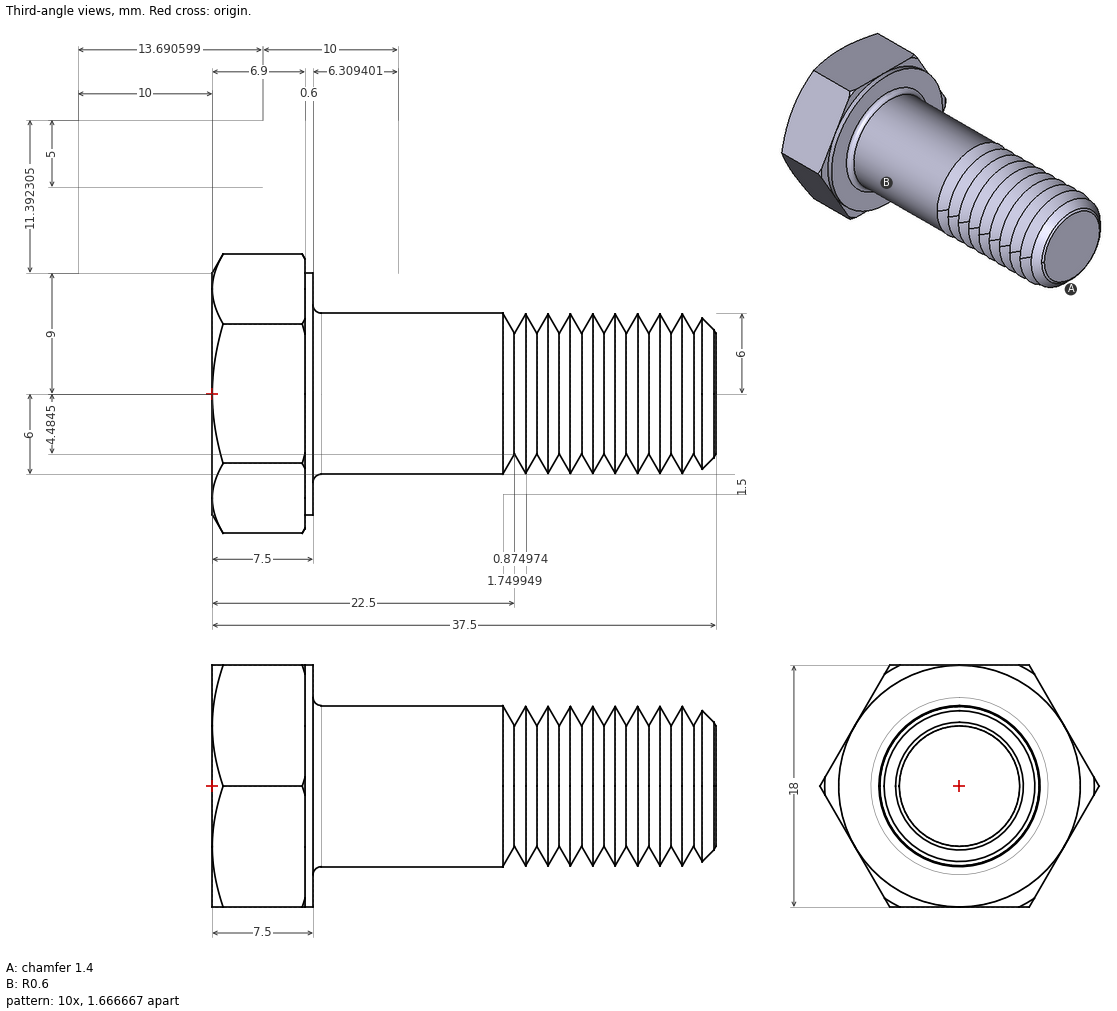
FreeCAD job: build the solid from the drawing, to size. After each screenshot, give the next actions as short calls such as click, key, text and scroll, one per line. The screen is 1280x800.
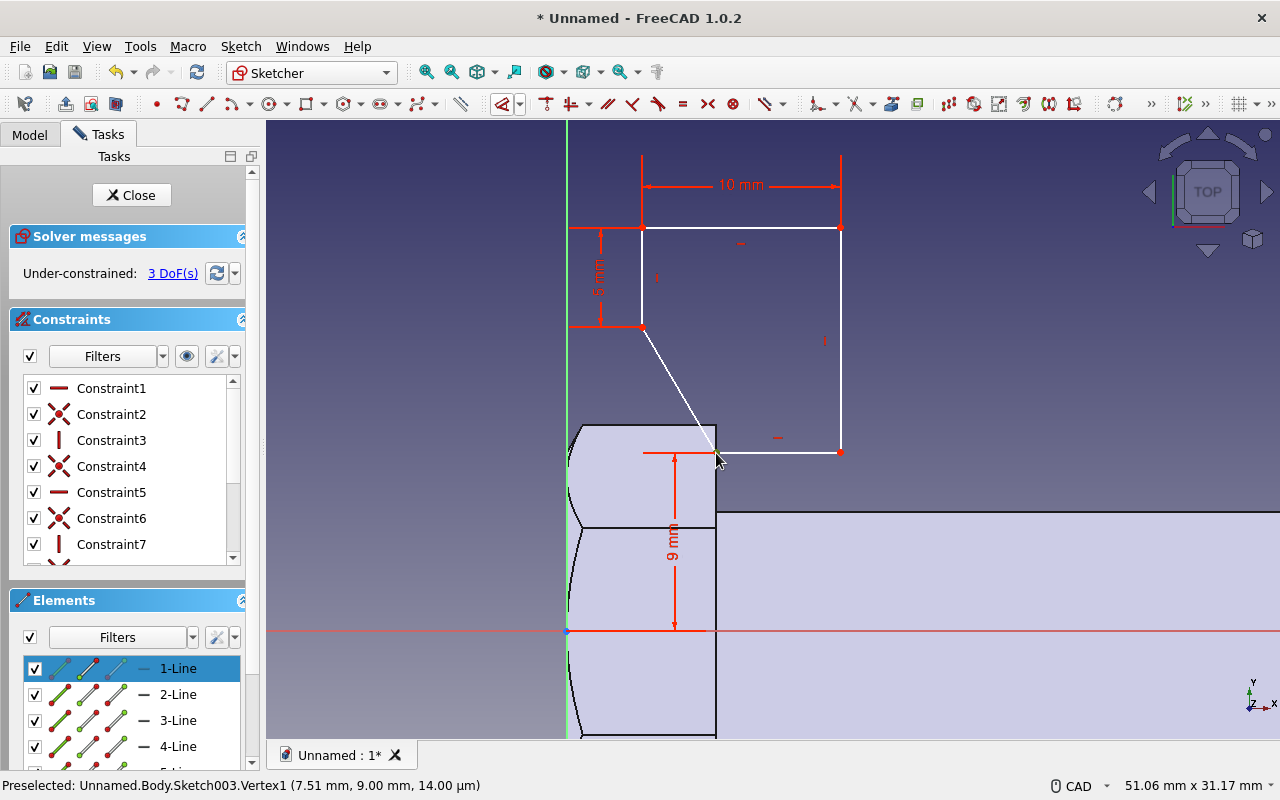
click(520, 104)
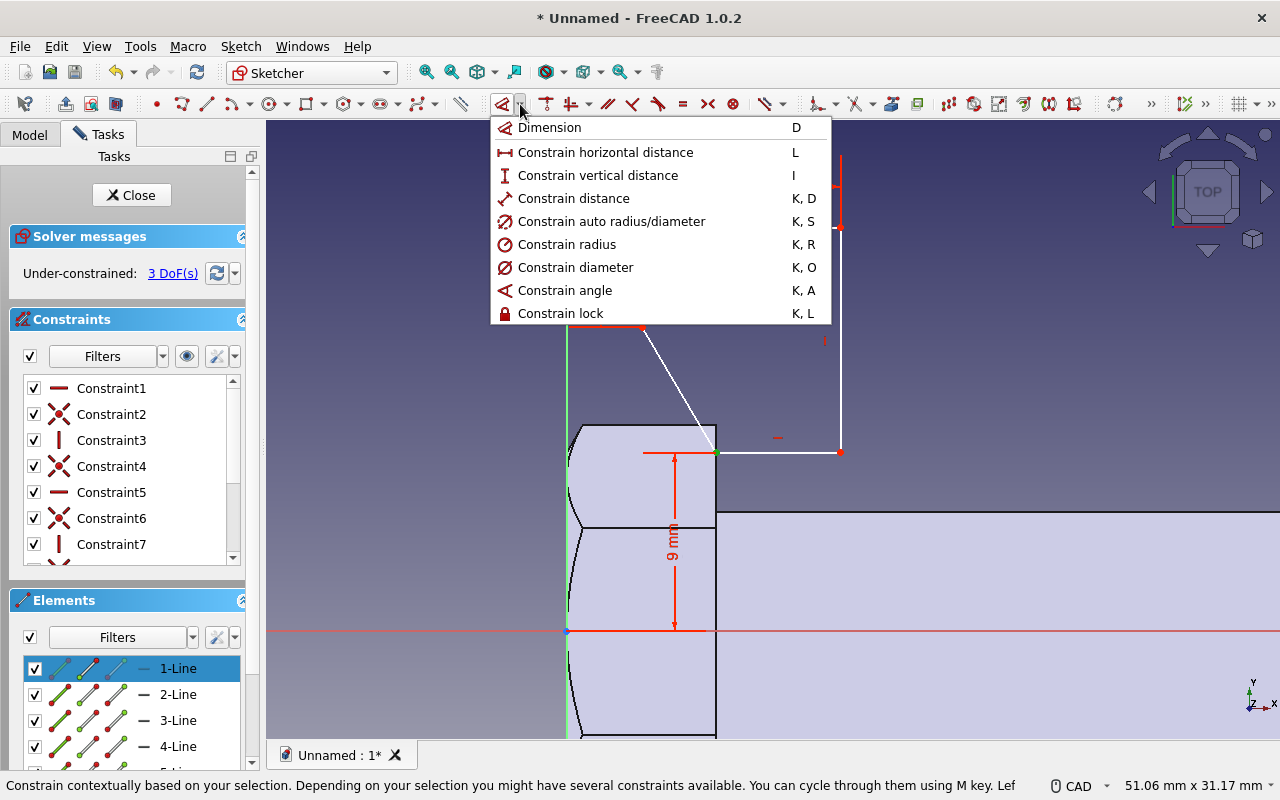
click(661, 152)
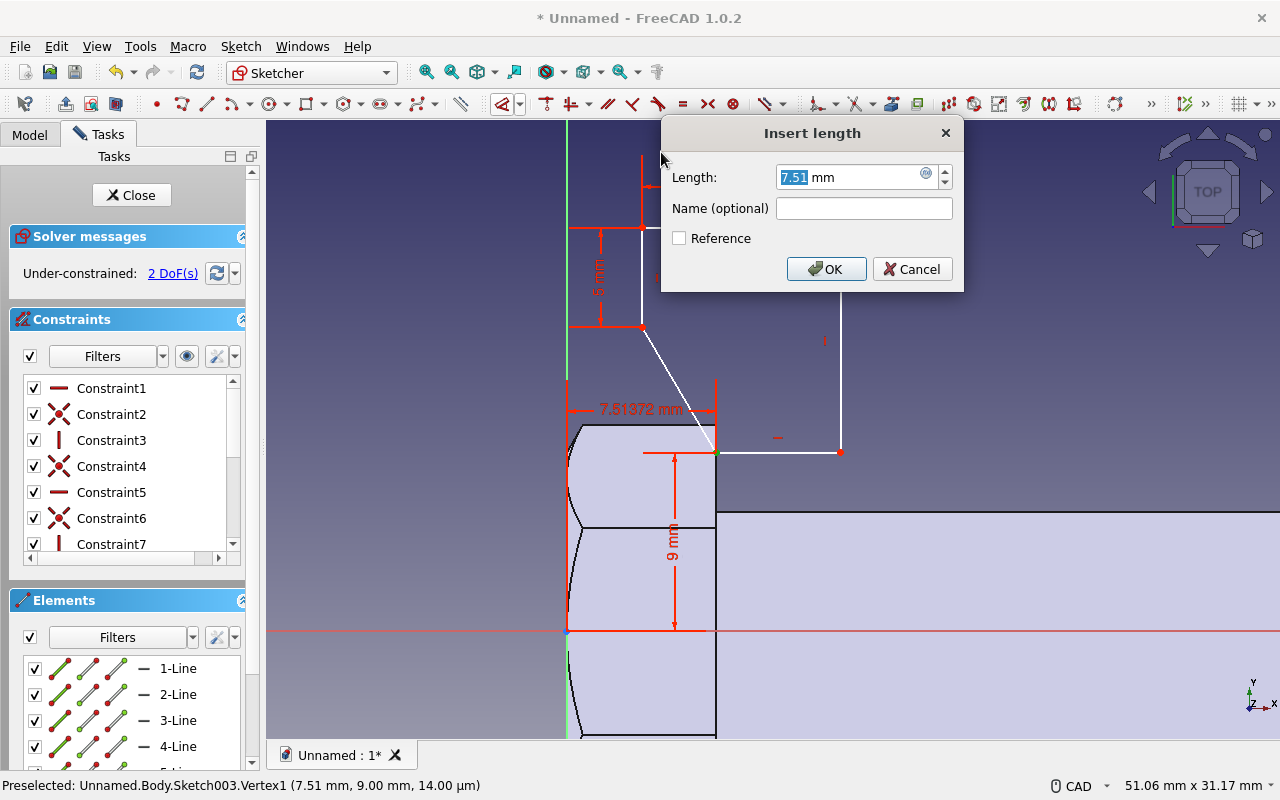
text(7.5)
key(Return)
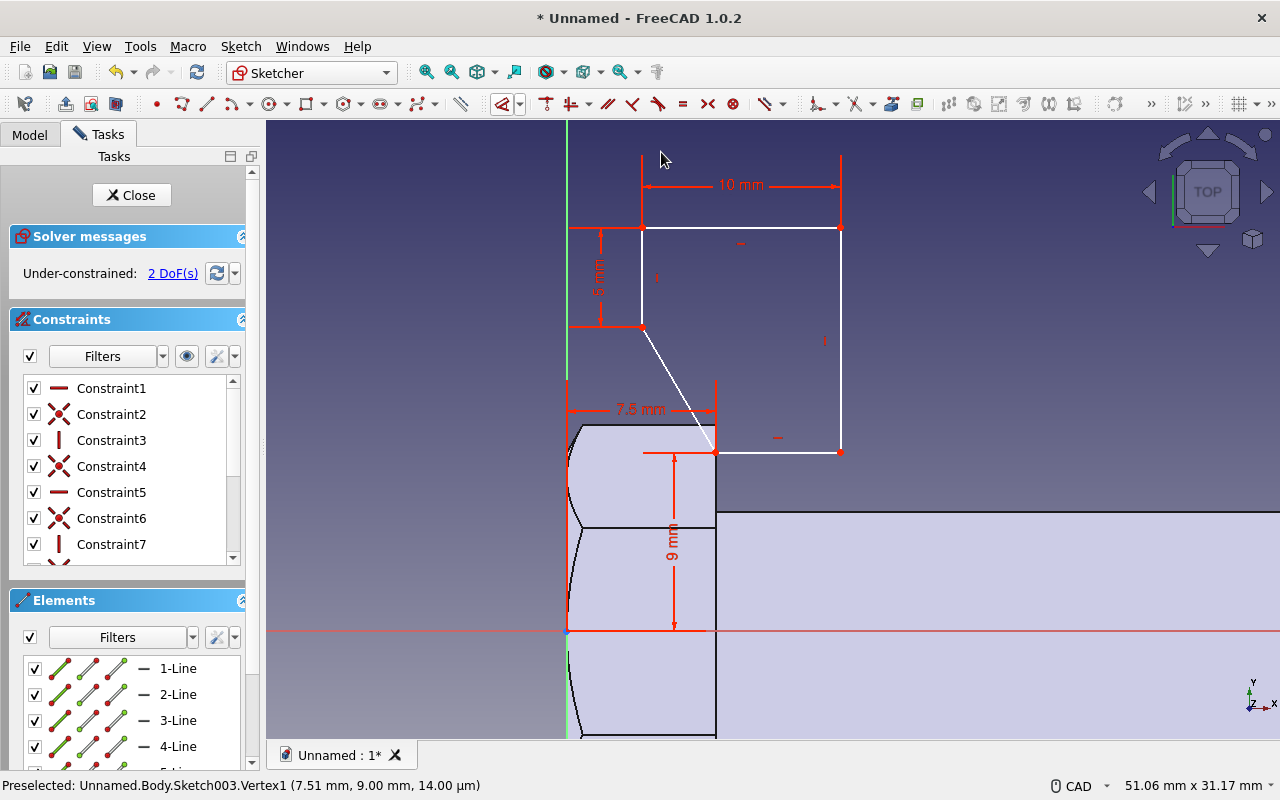
click(753, 453)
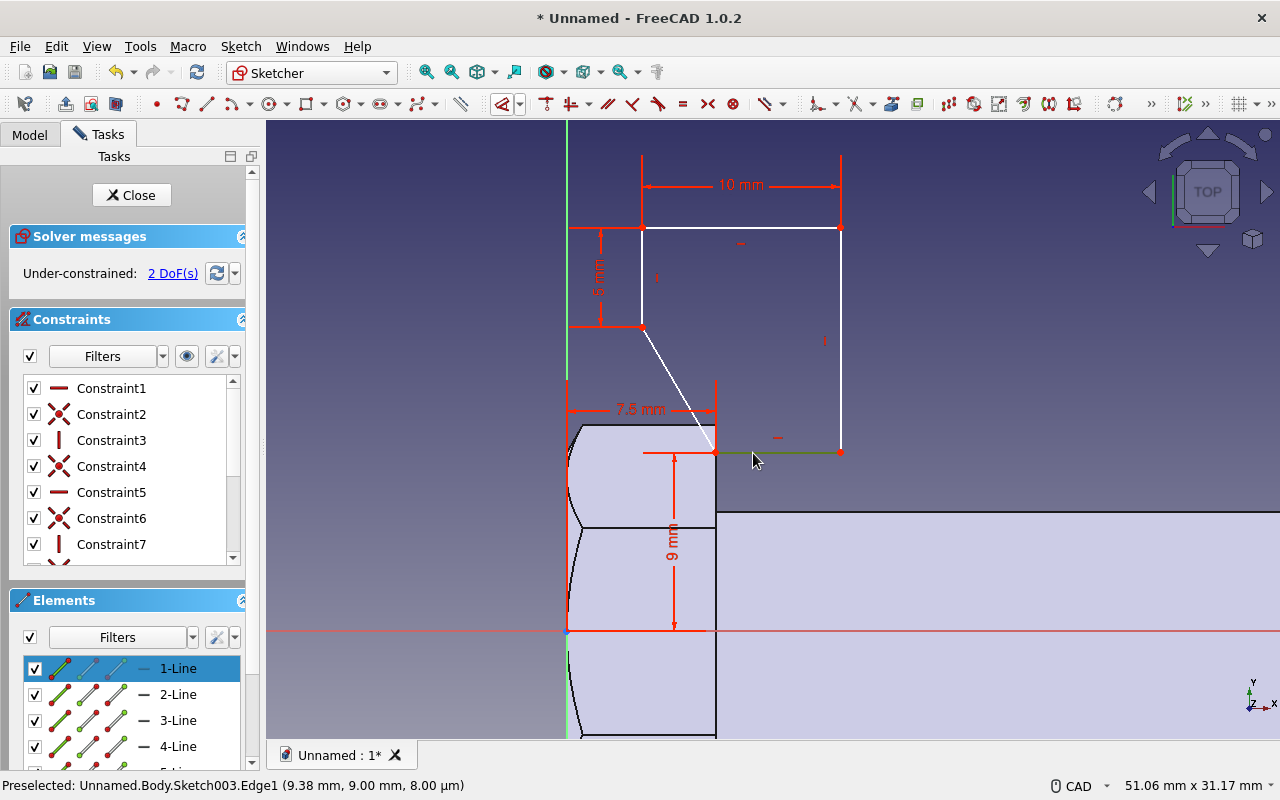
click(520, 104)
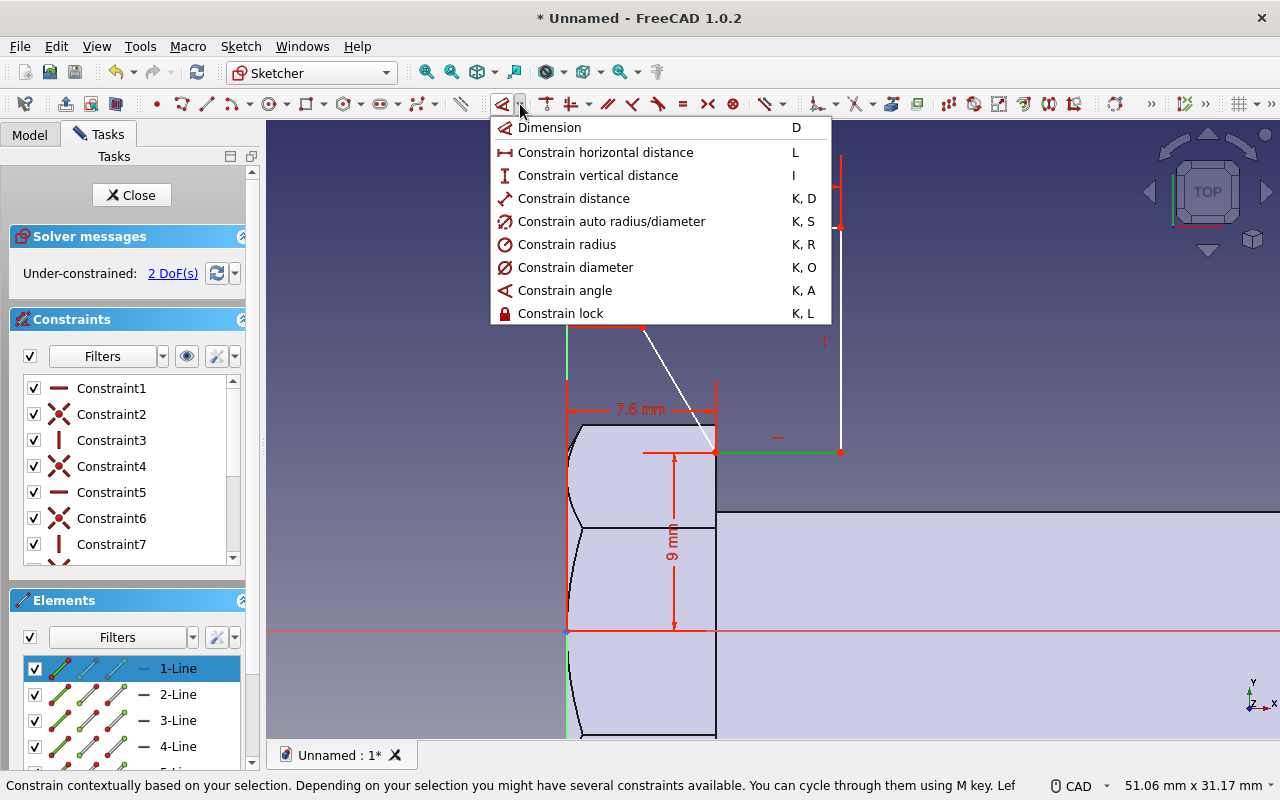
click(661, 152)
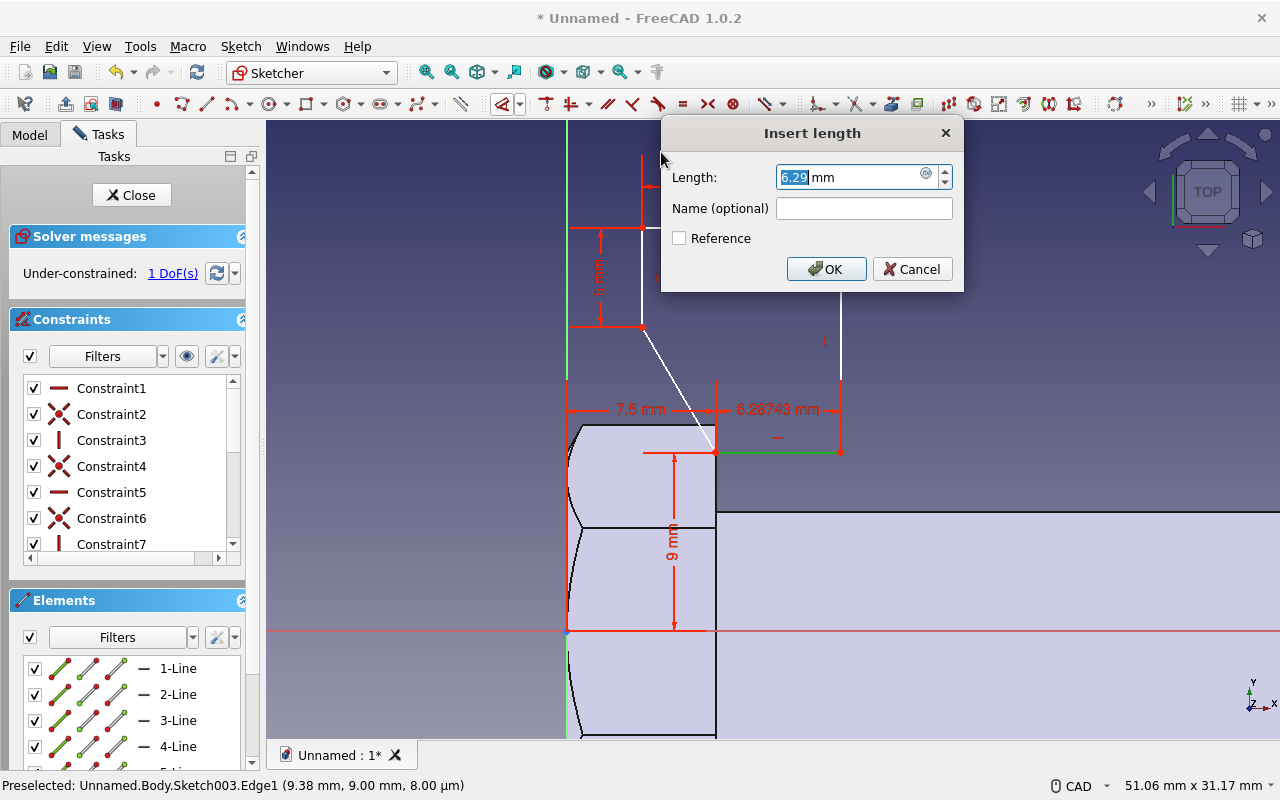
text(6.309401)
key(Return)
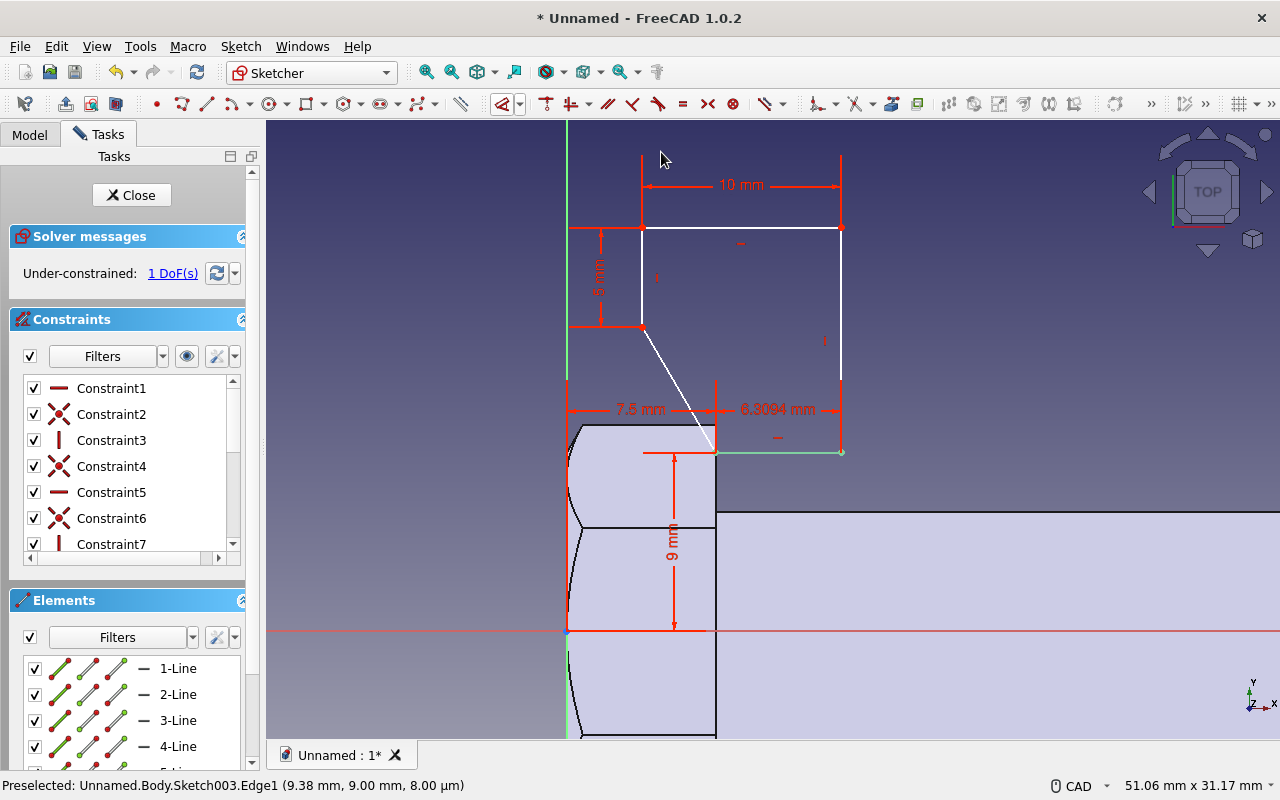
click(841, 385)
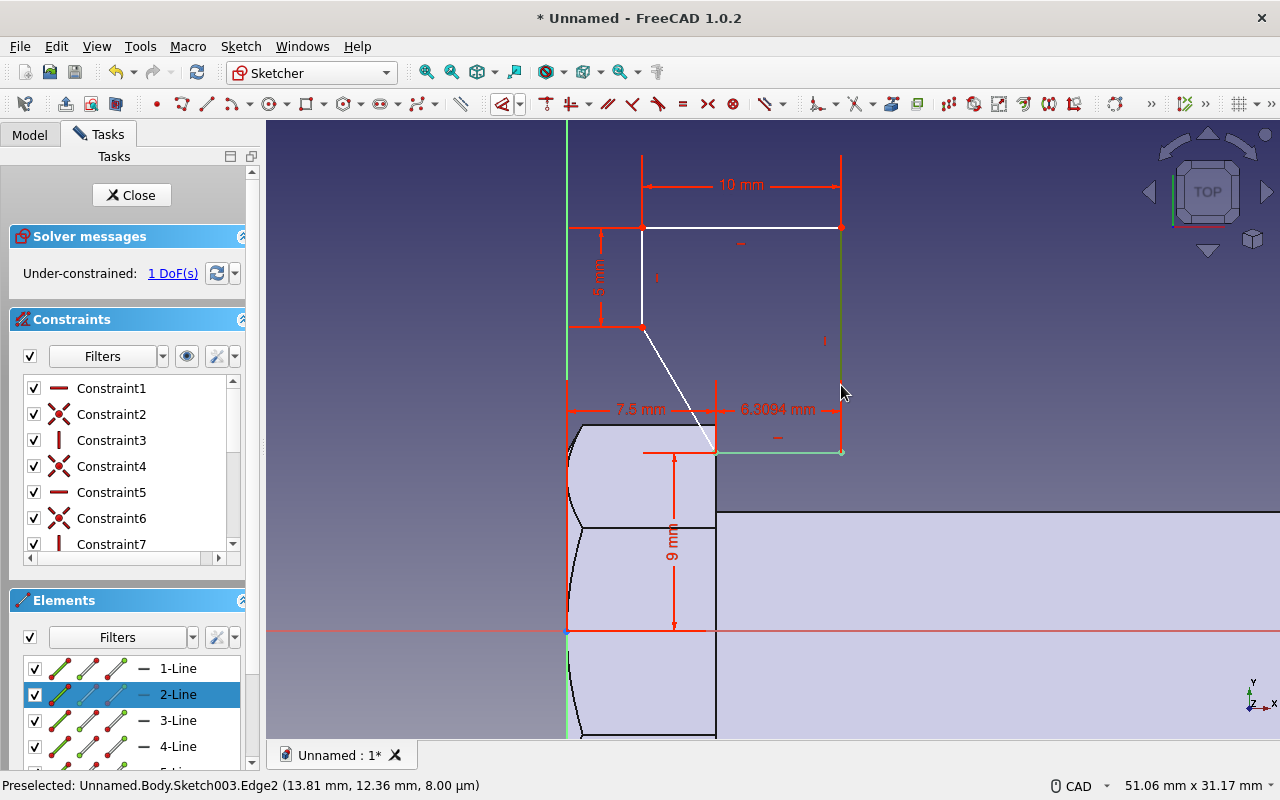
click(520, 104)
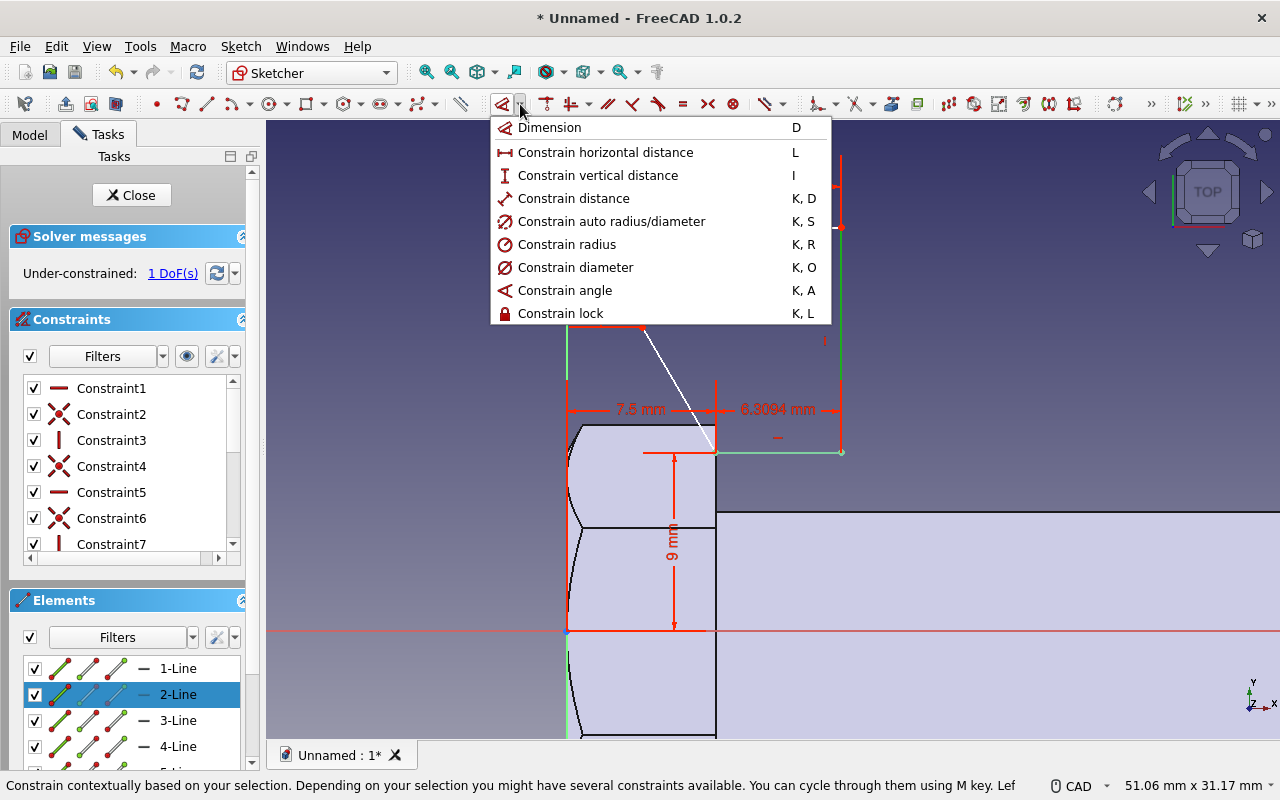
click(661, 176)